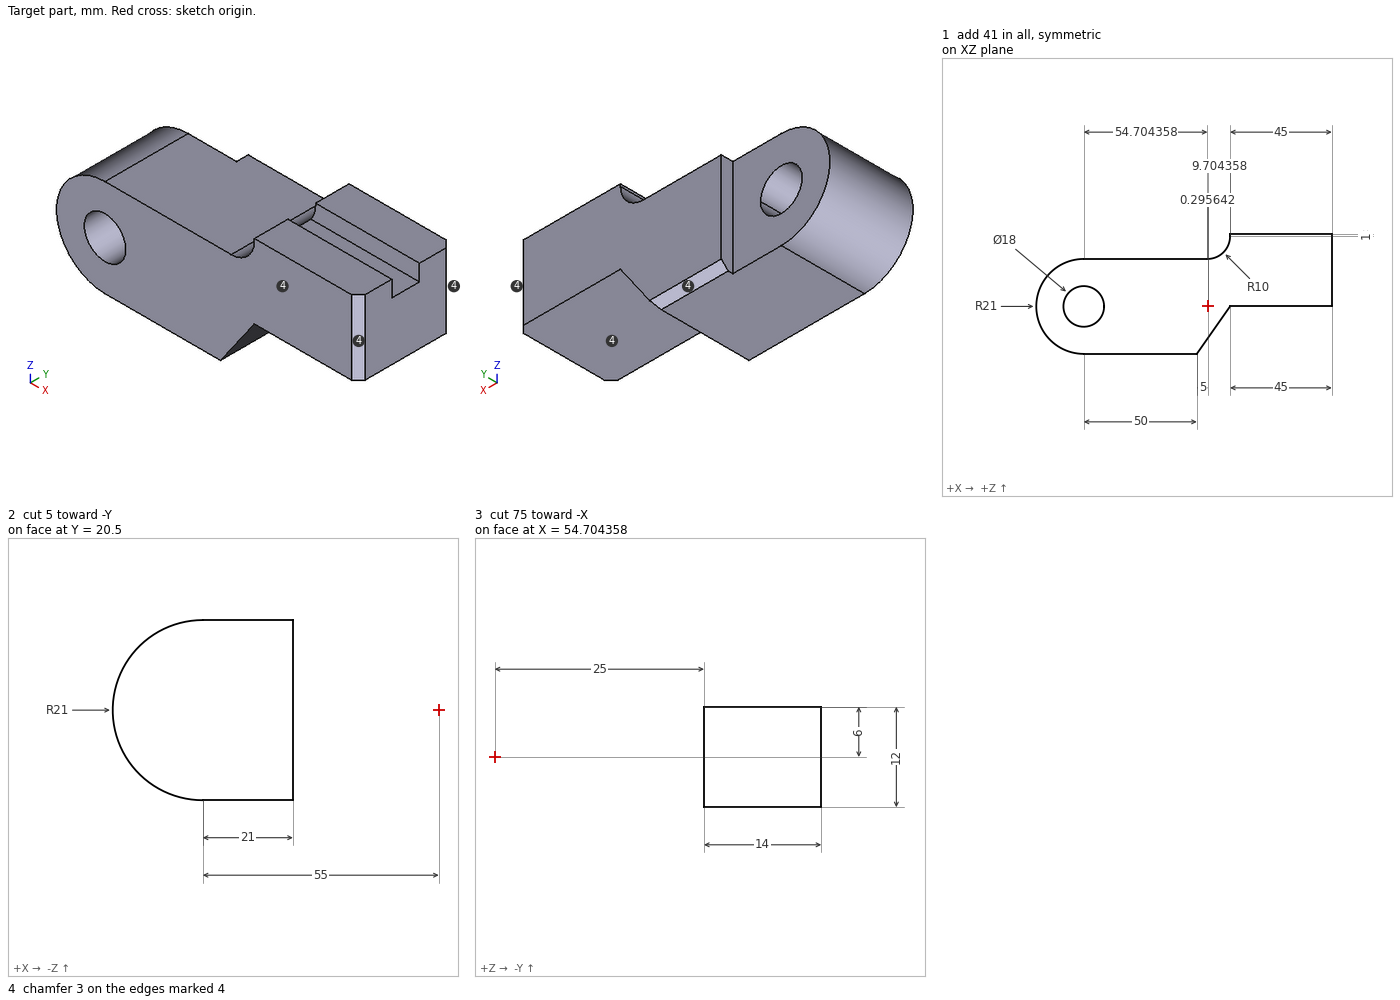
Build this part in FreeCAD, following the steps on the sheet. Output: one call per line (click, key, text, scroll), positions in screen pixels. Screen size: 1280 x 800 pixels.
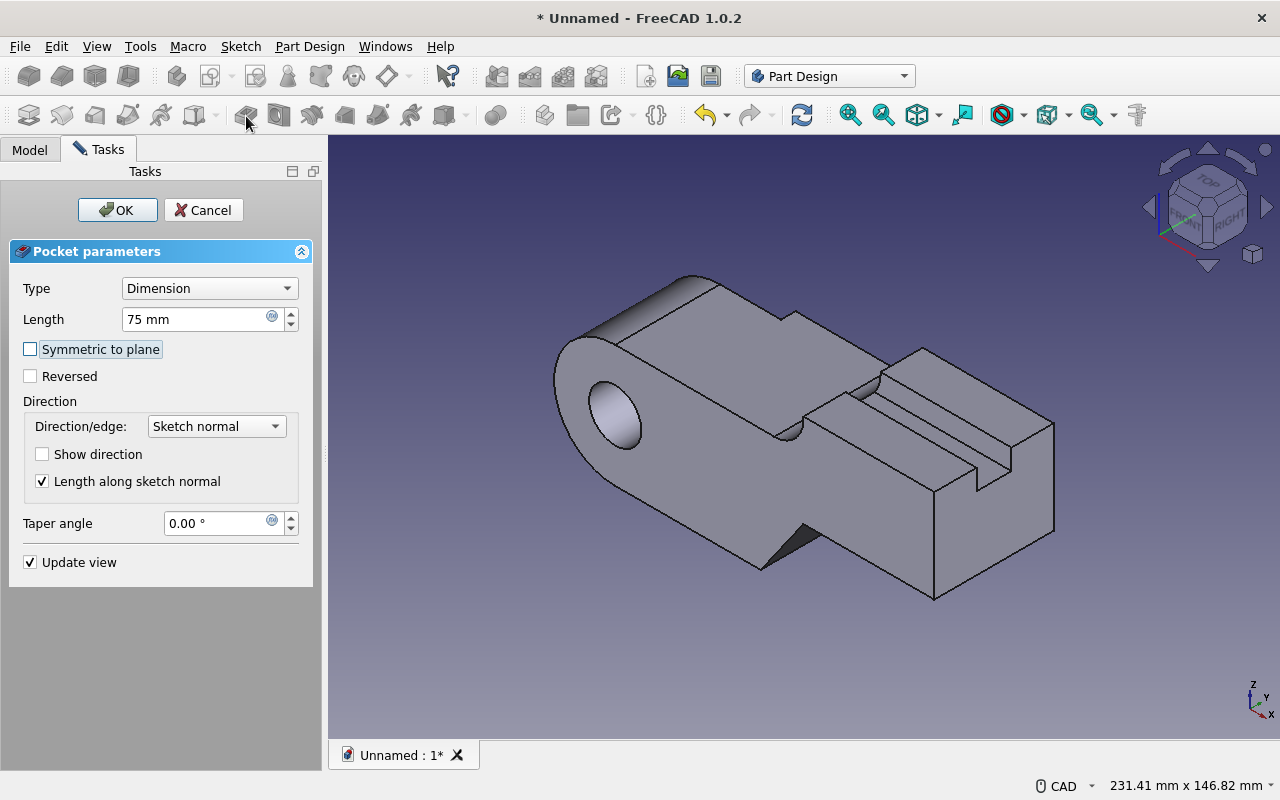
click(118, 210)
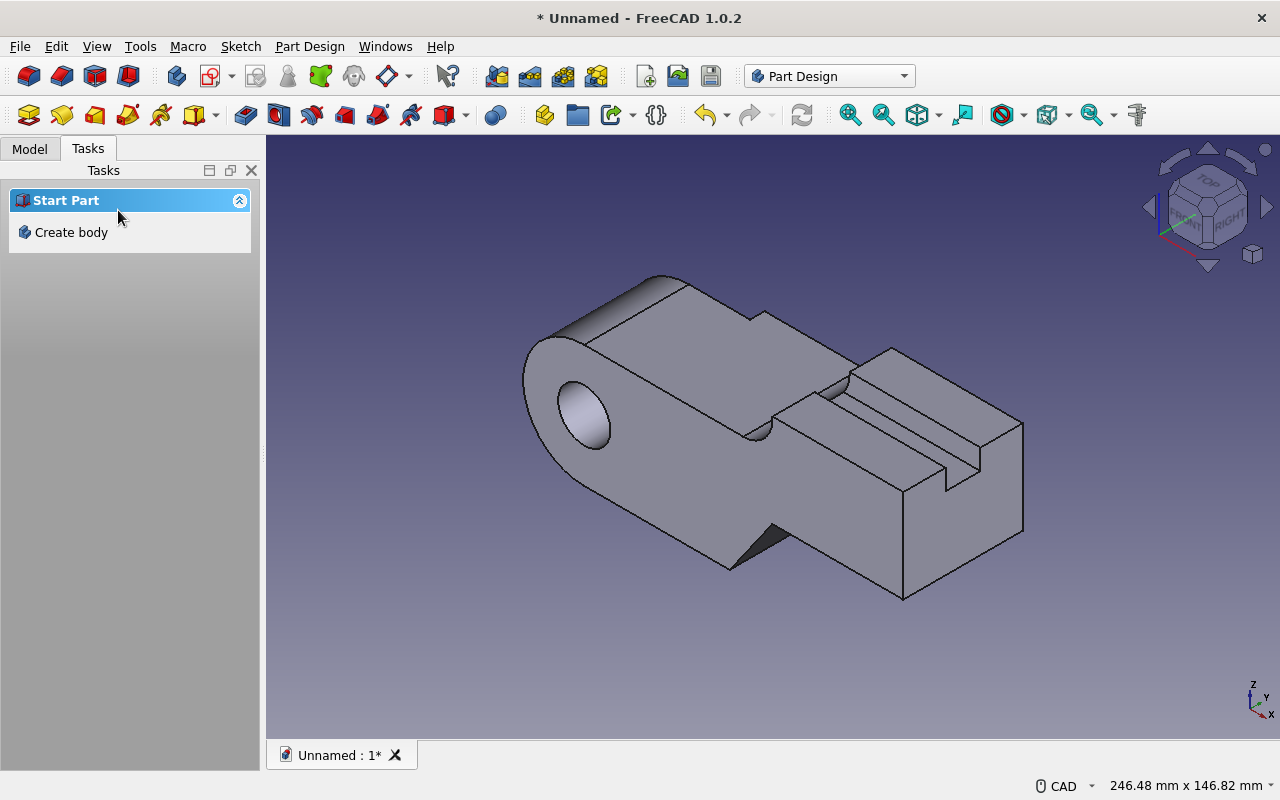
click(903, 545)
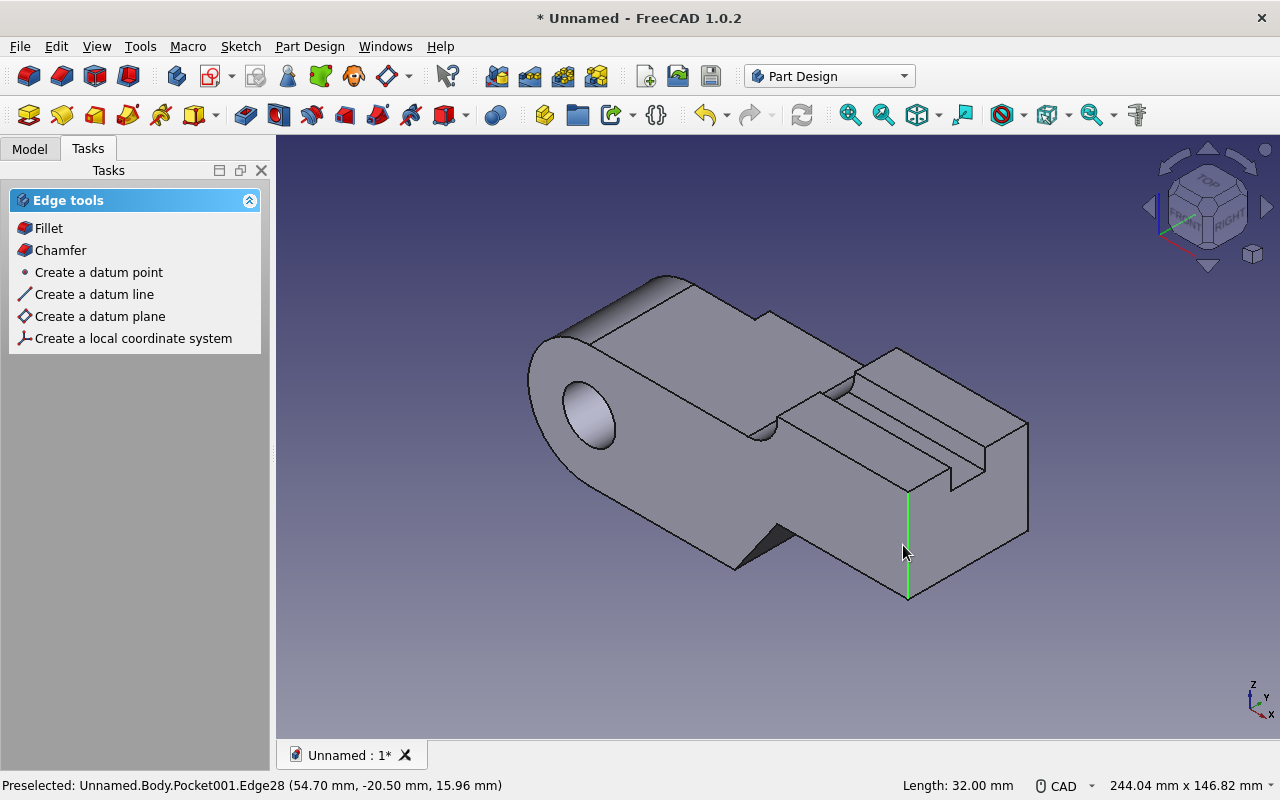
key(2)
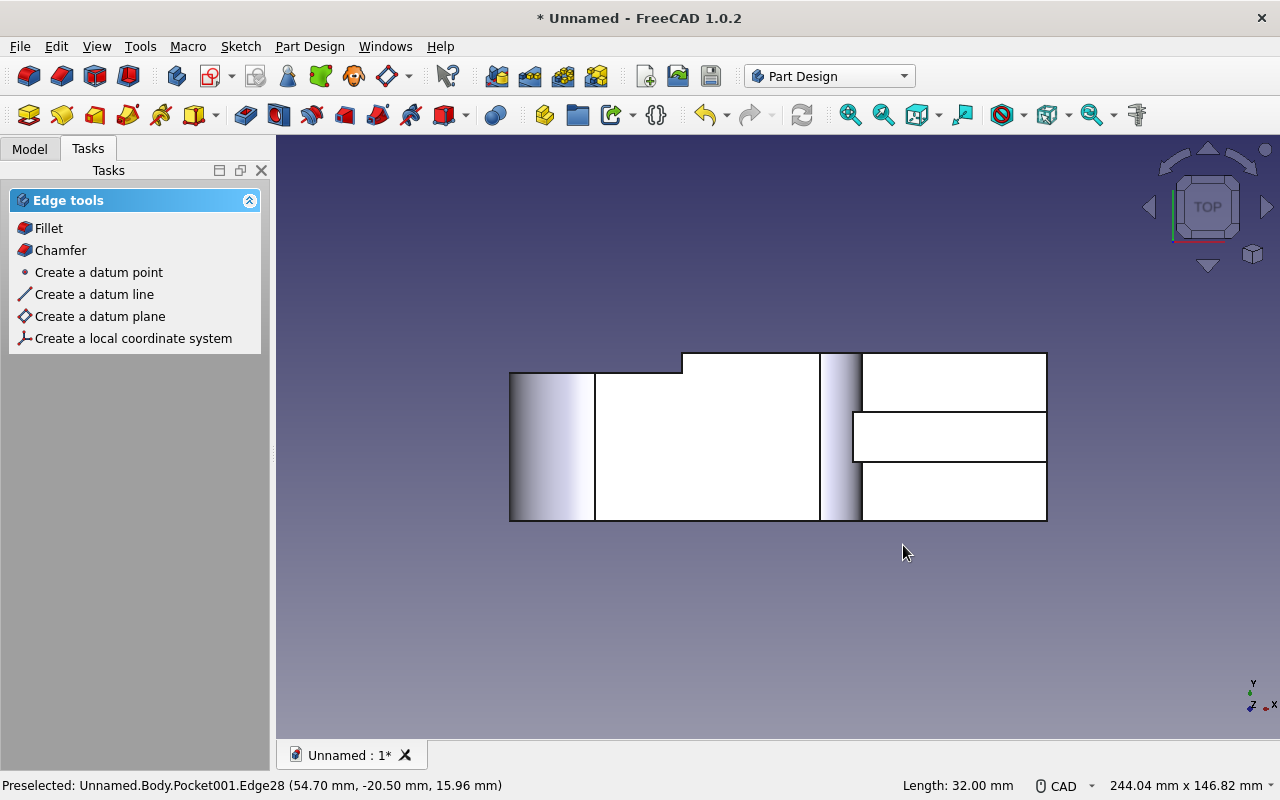
key(0)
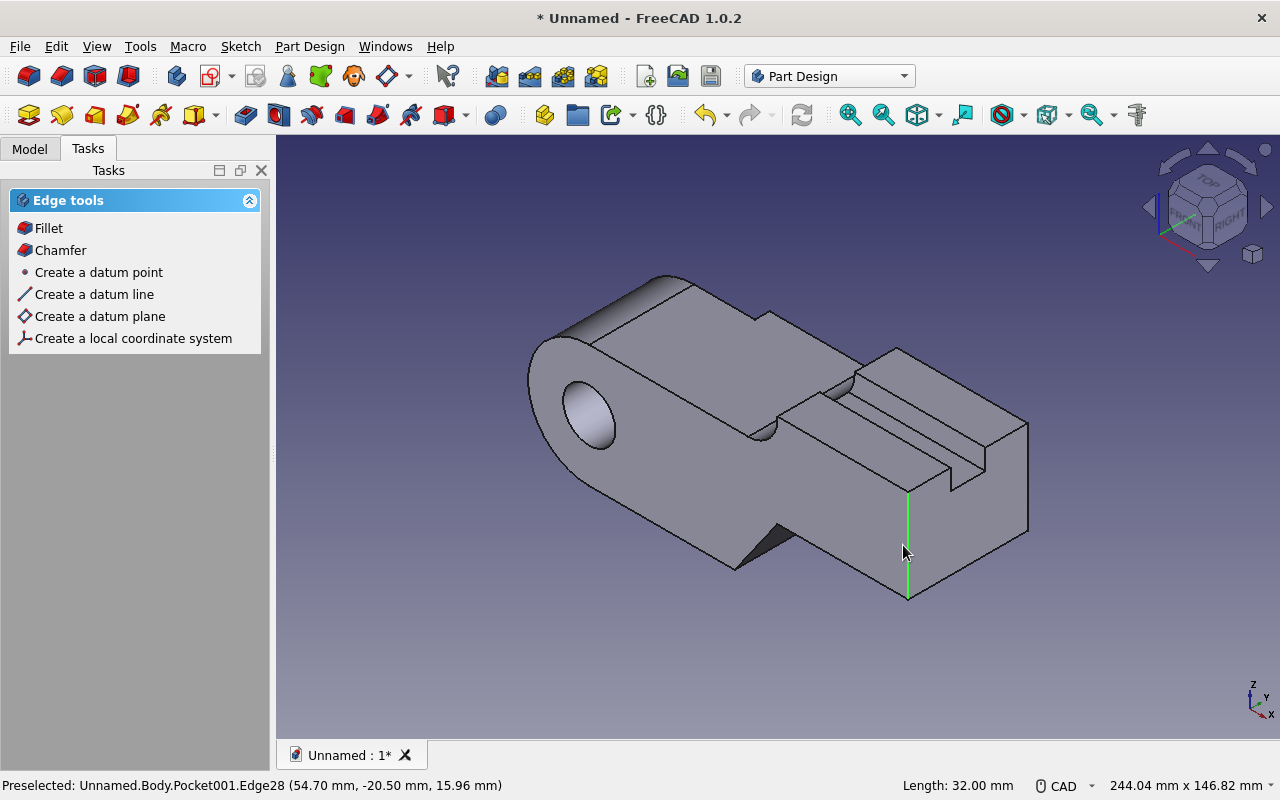
key(1)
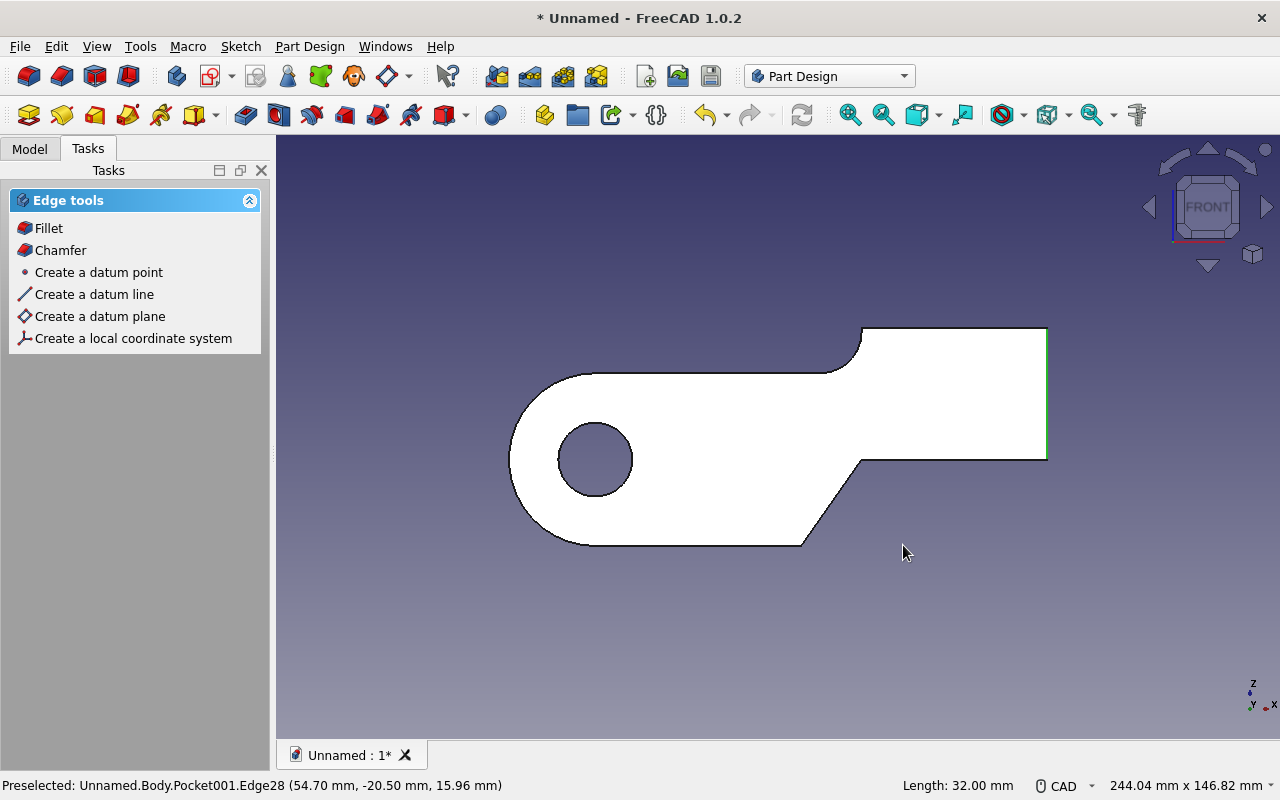
key(3)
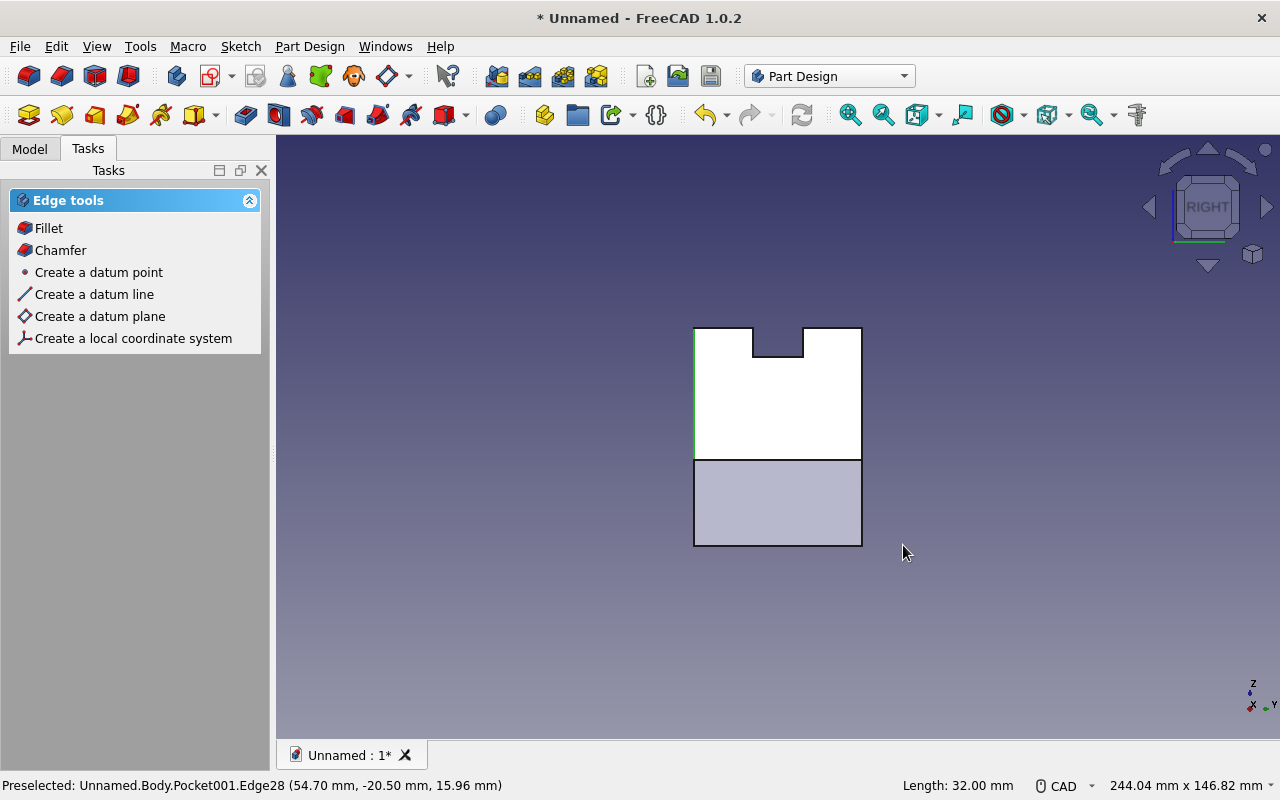
key(v)
key(f)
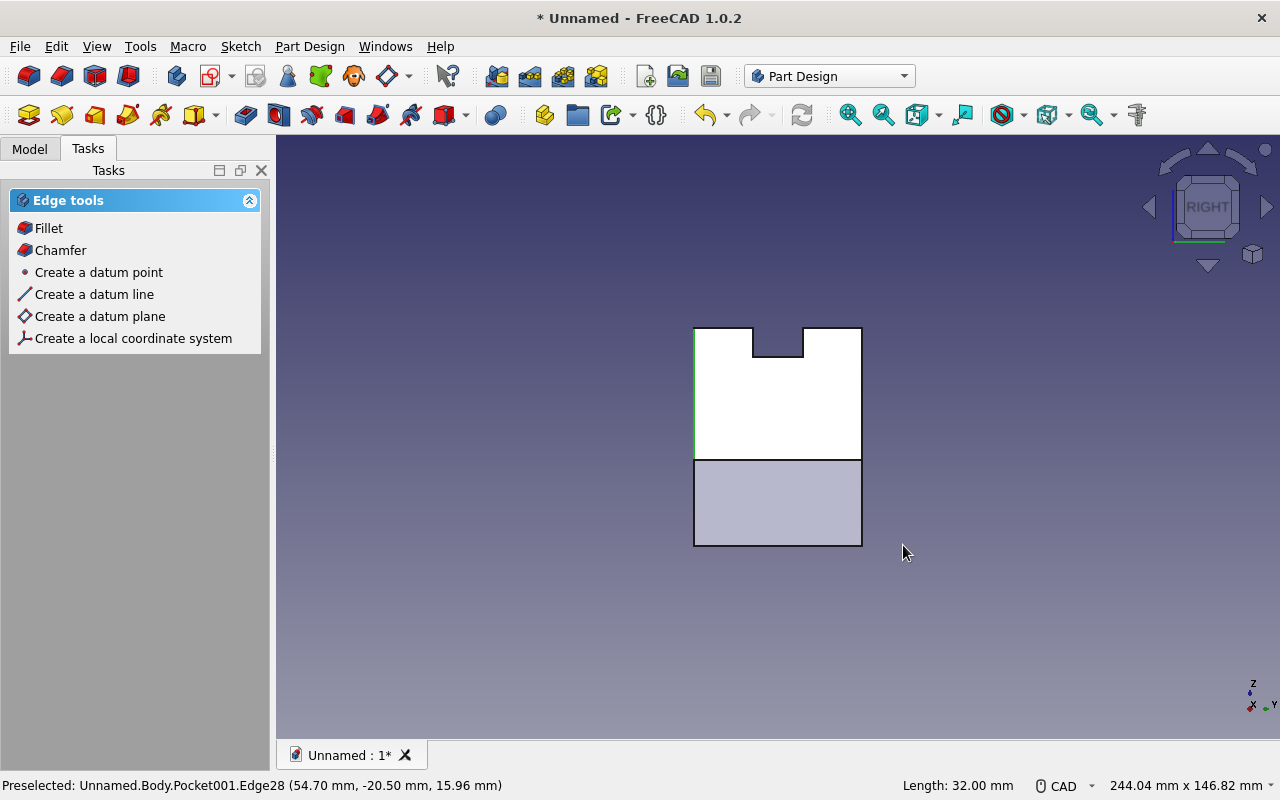
click(862, 393, ctrl)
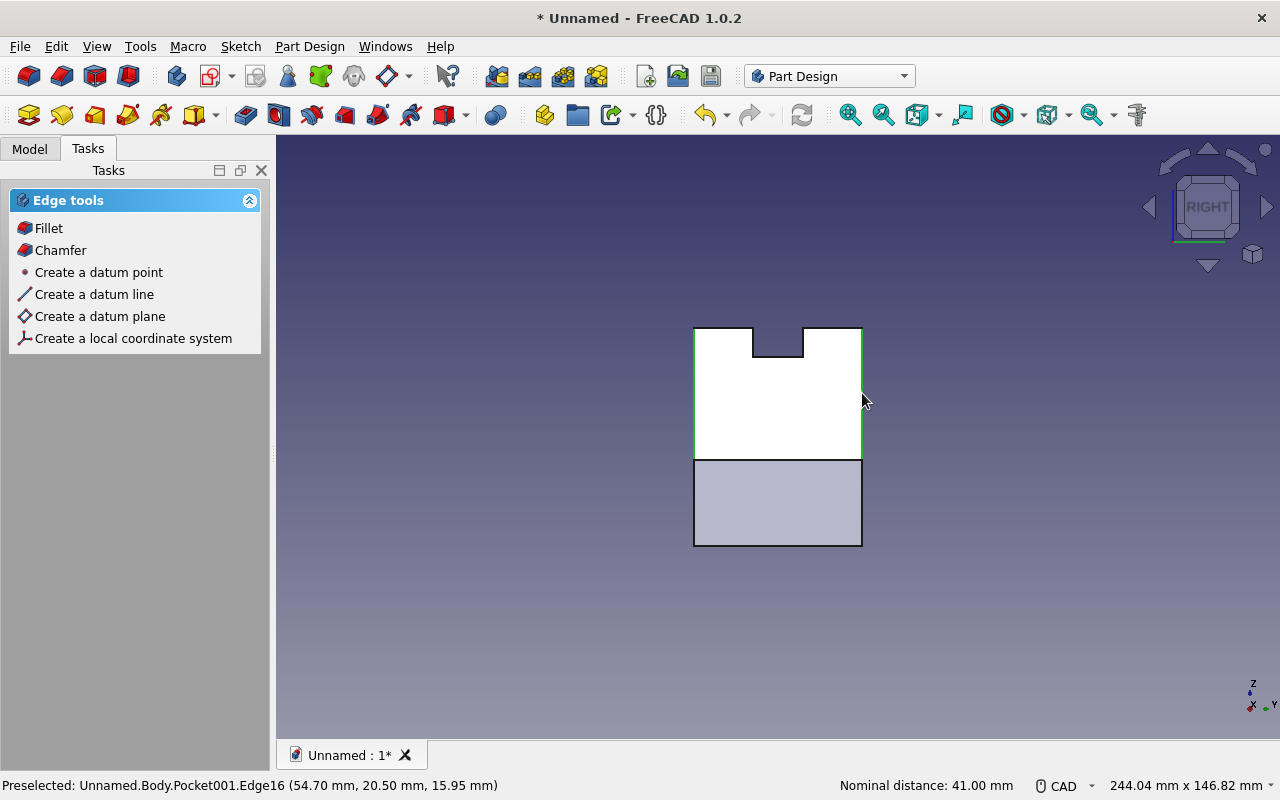
key(5)